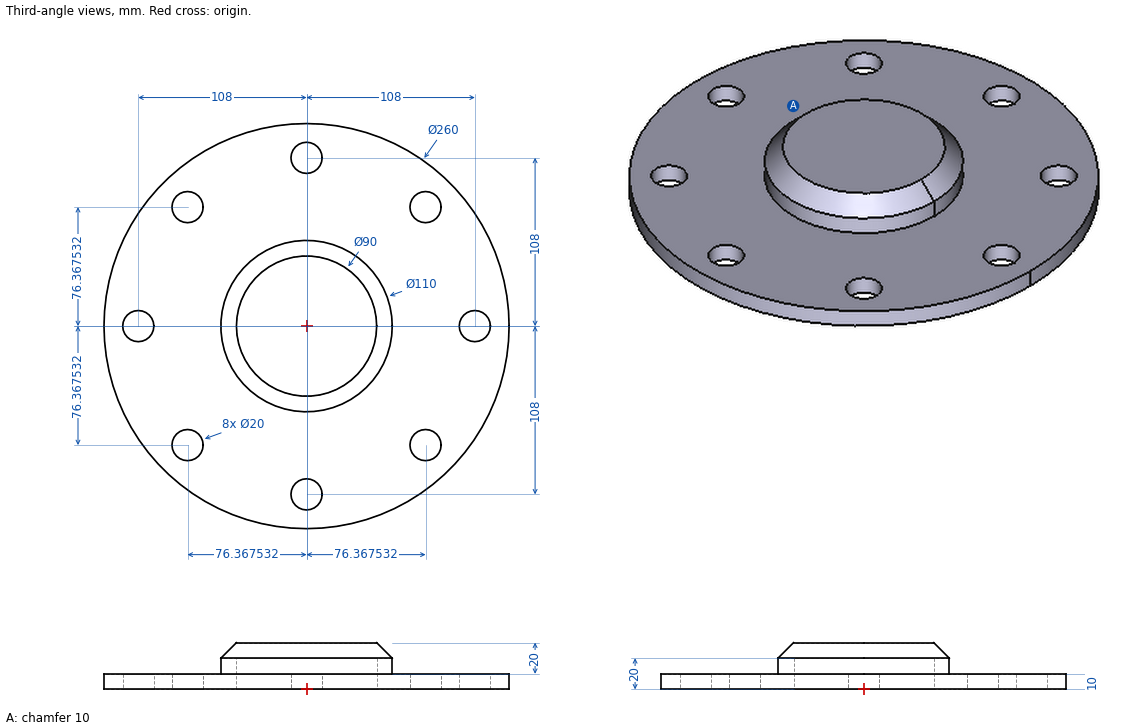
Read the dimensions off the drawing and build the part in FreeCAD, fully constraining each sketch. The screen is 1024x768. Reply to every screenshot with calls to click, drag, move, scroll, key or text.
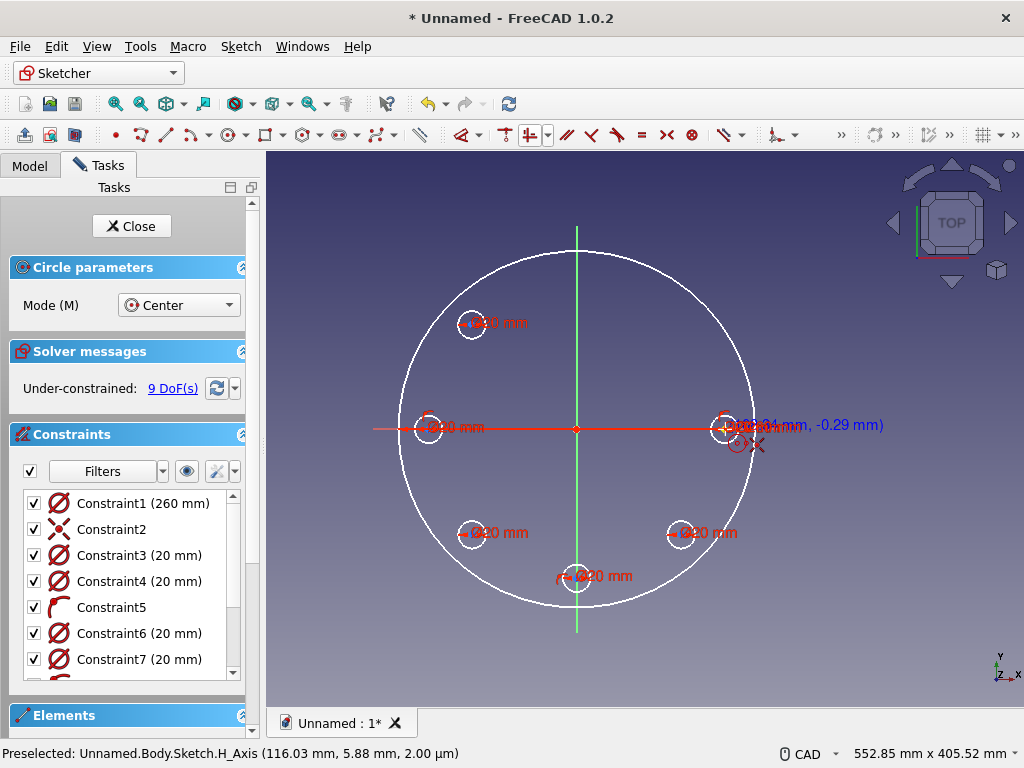
scroll(577, 281, up, 3)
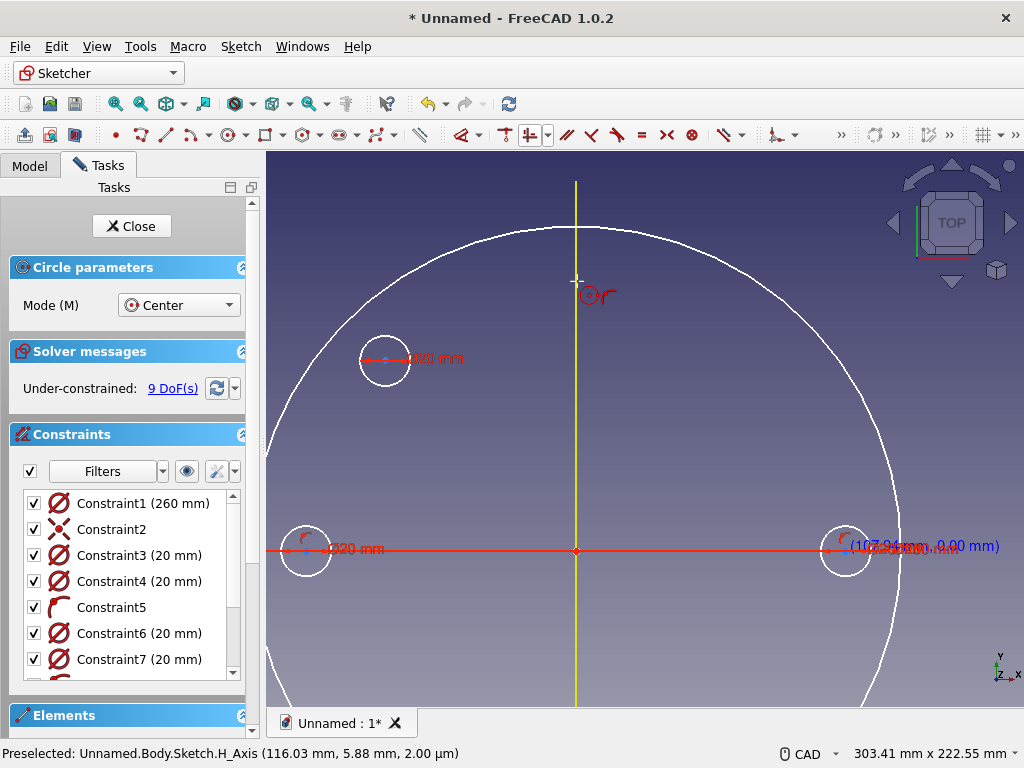
click(576, 281)
move(594, 264)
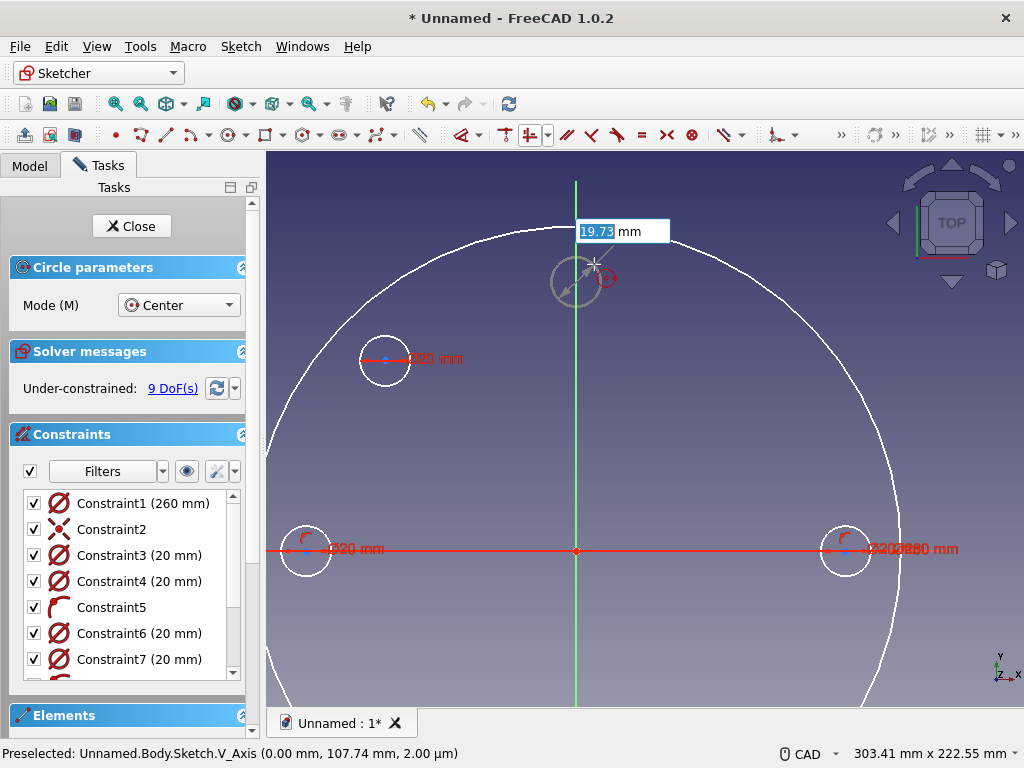
text(20)
key(Return)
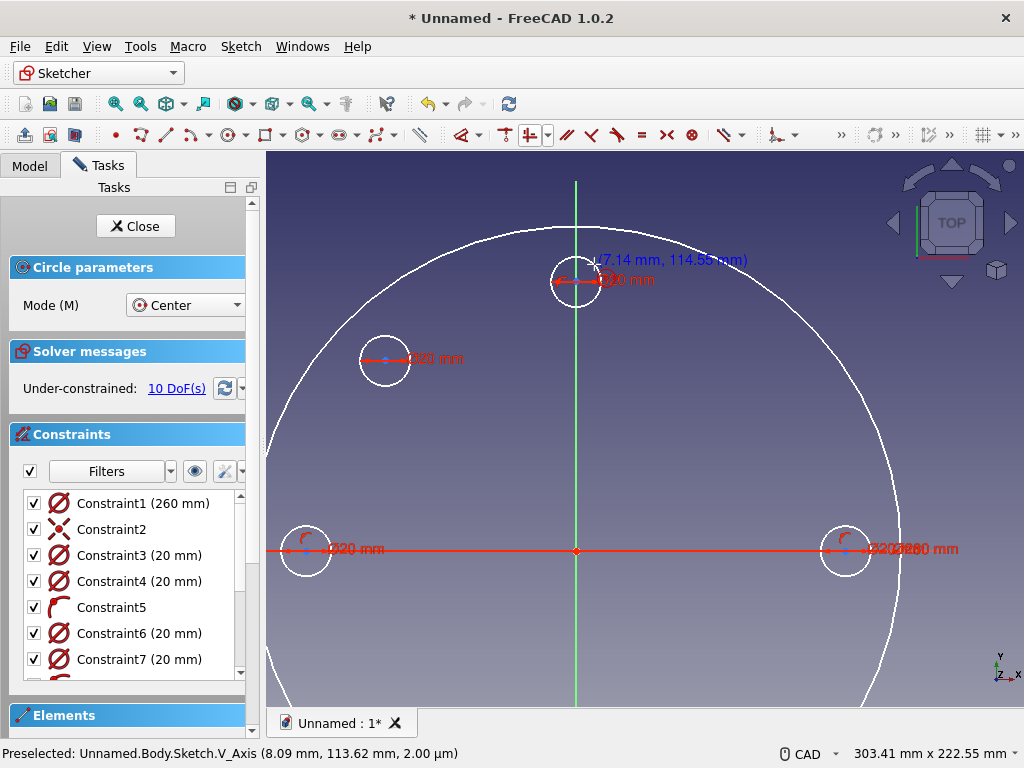
click(767, 360)
move(785, 343)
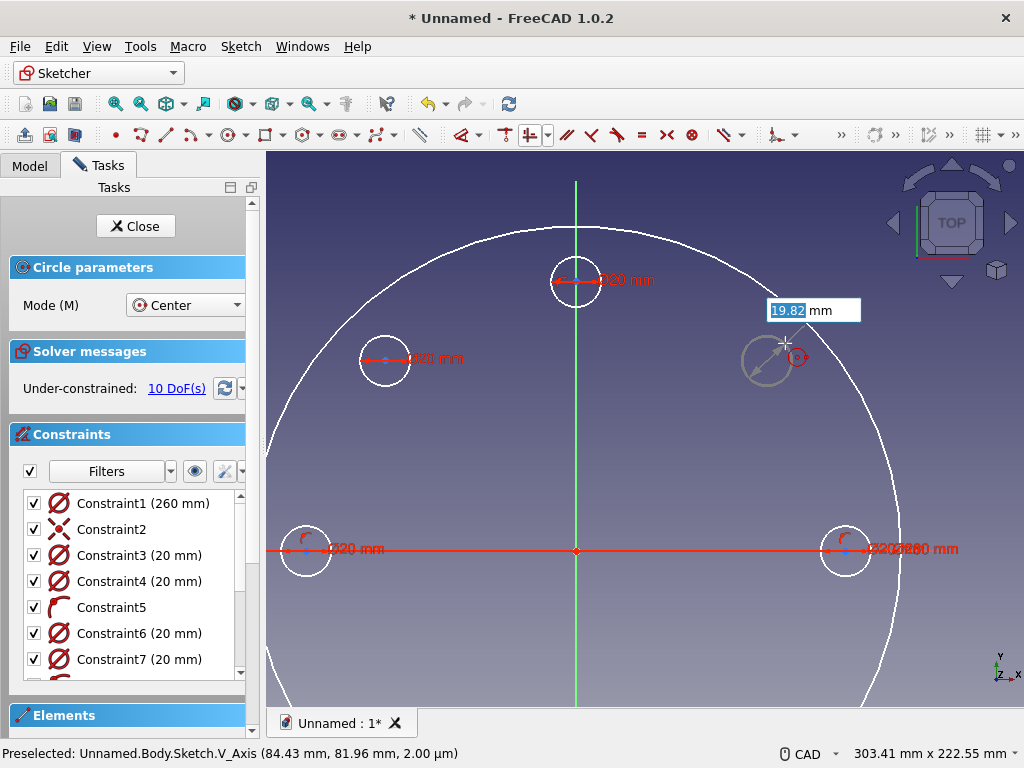
text(20)
key(Return)
key(Escape)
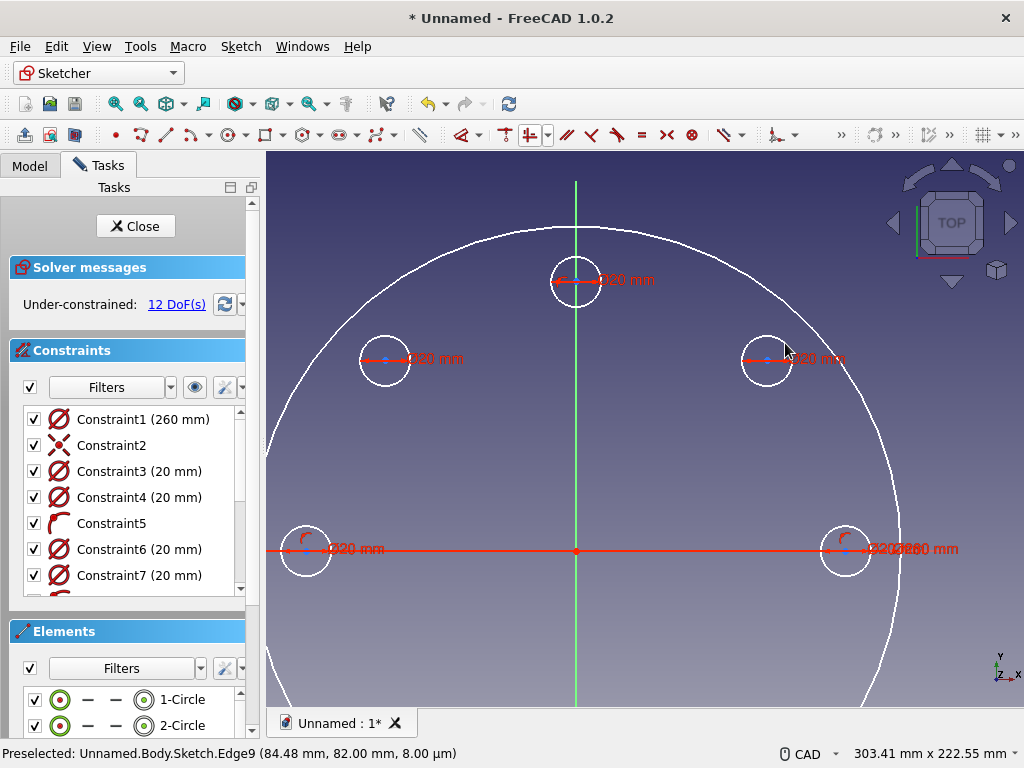
key(d)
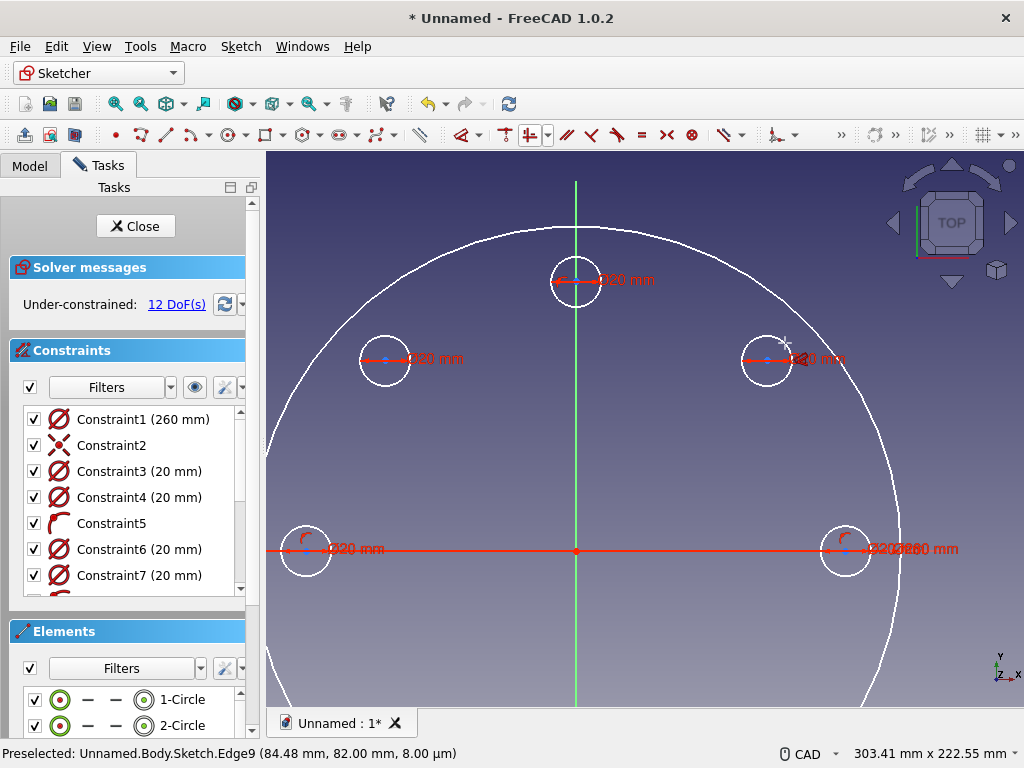
scroll(577, 280, down, 3)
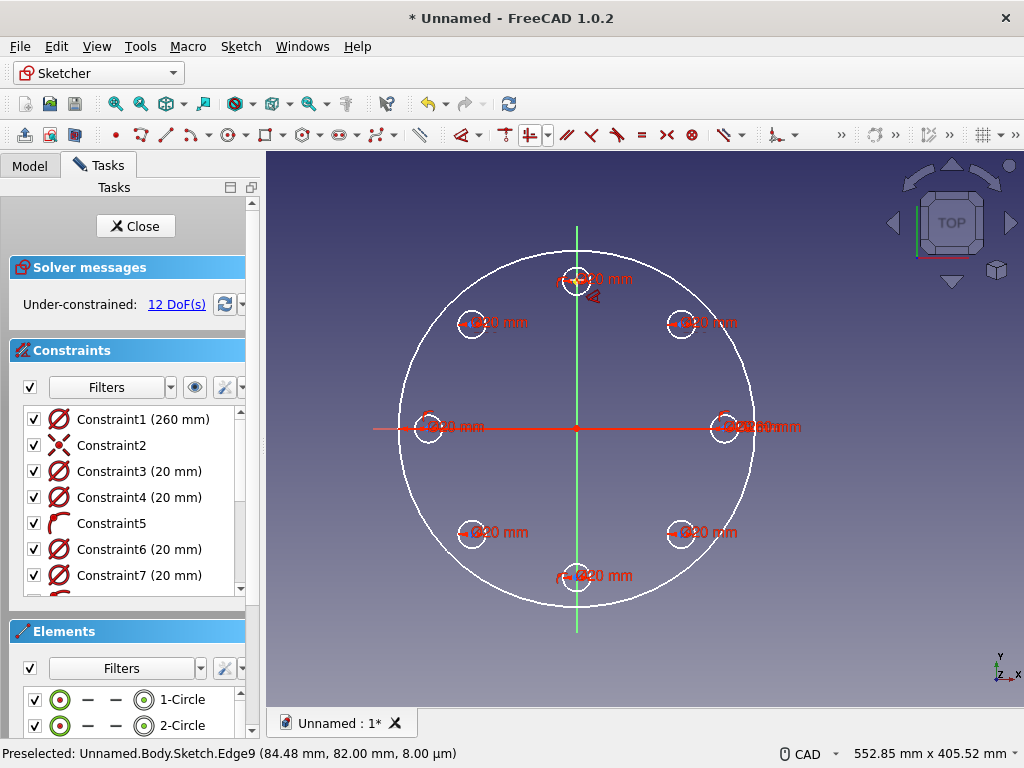
click(577, 578)
click(611, 503)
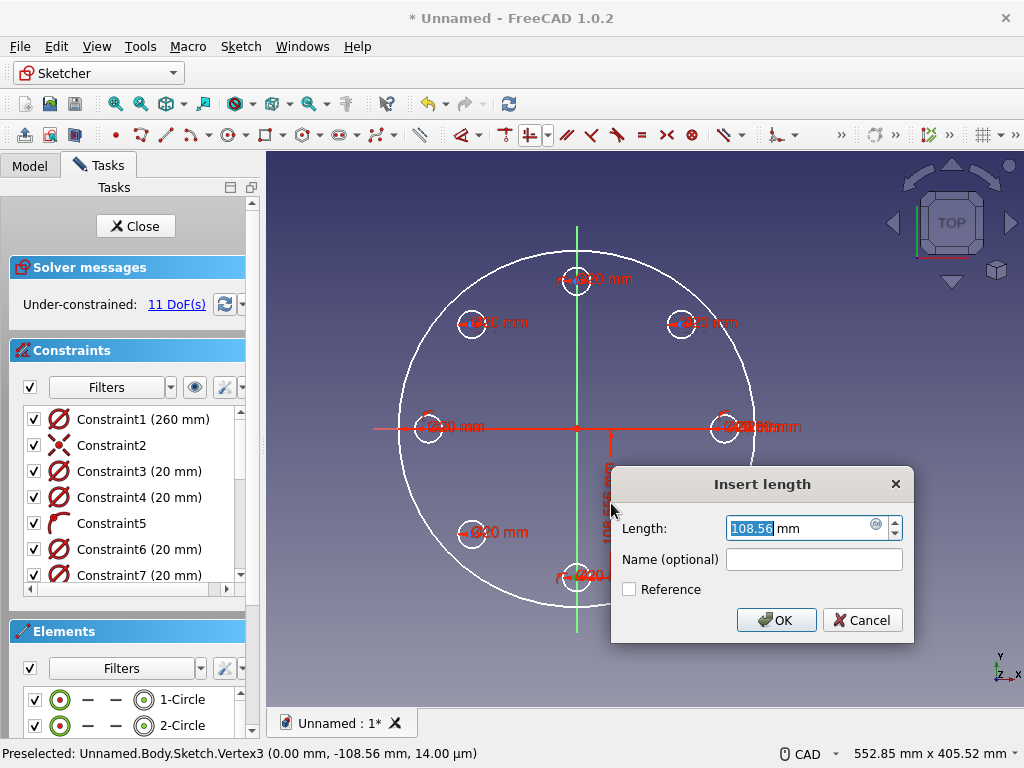
text(108)
key(Return)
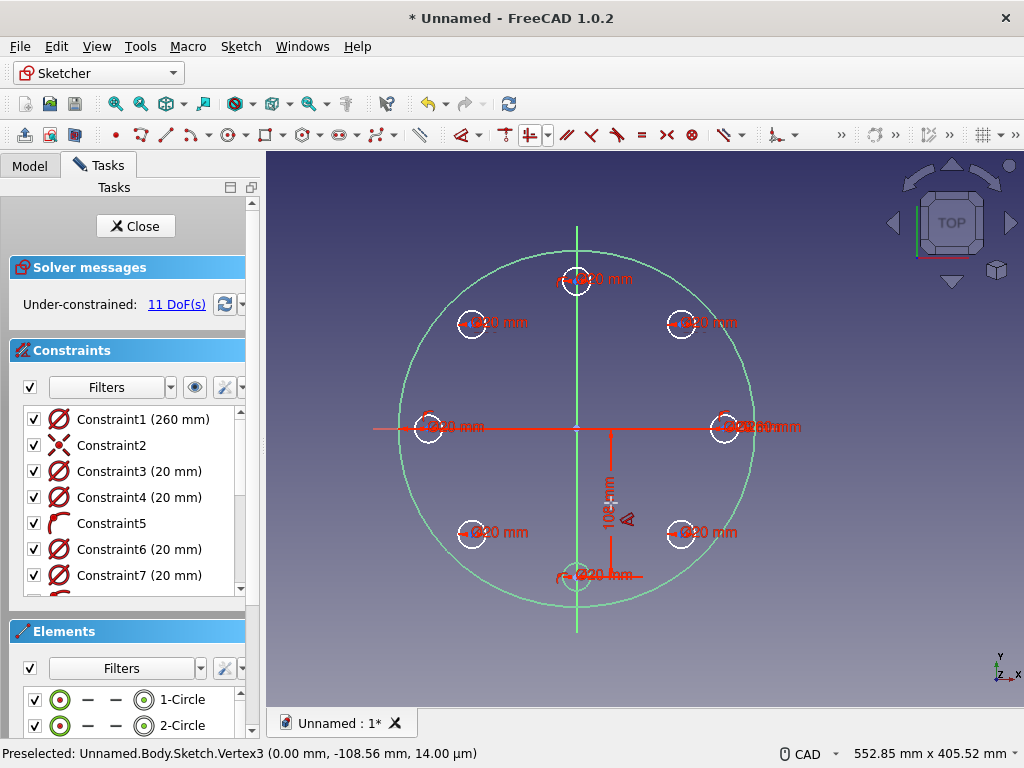
click(429, 429)
click(503, 463)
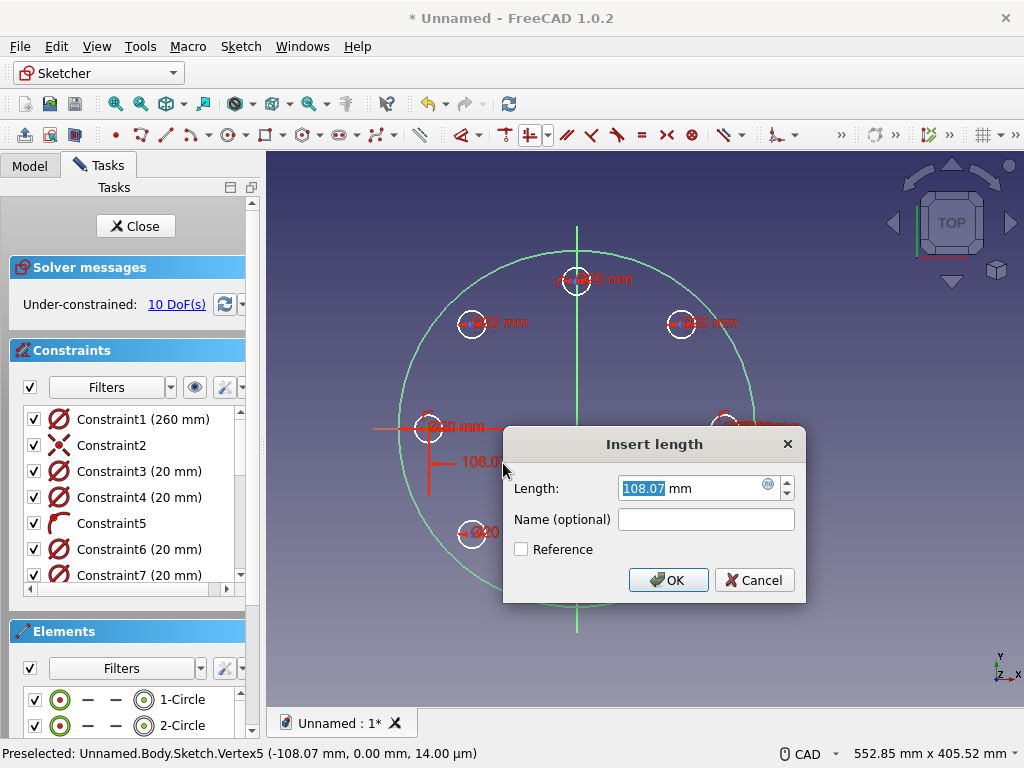
text(108)
key(Return)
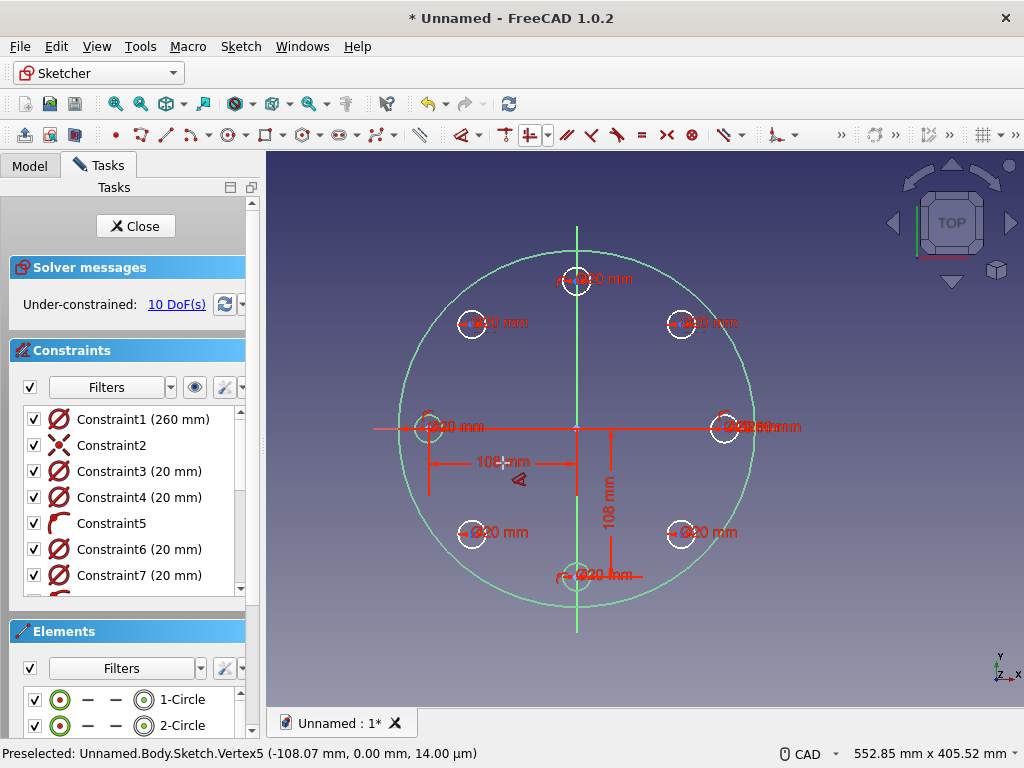
click(725, 429)
click(651, 463)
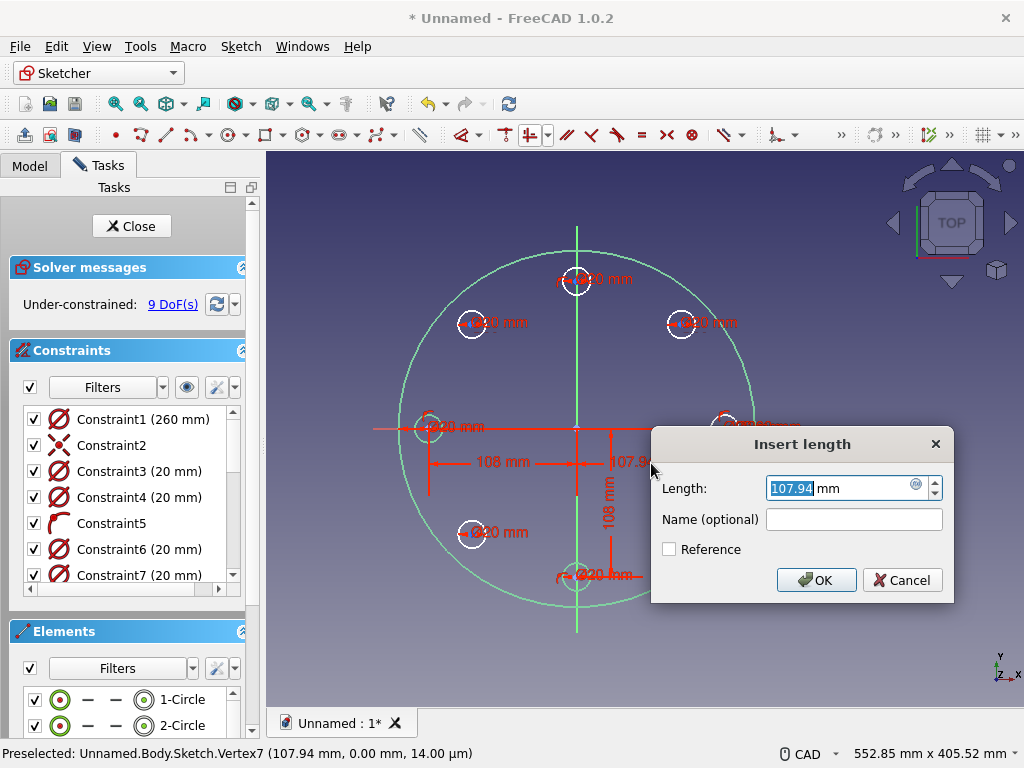
text(108)
key(Return)